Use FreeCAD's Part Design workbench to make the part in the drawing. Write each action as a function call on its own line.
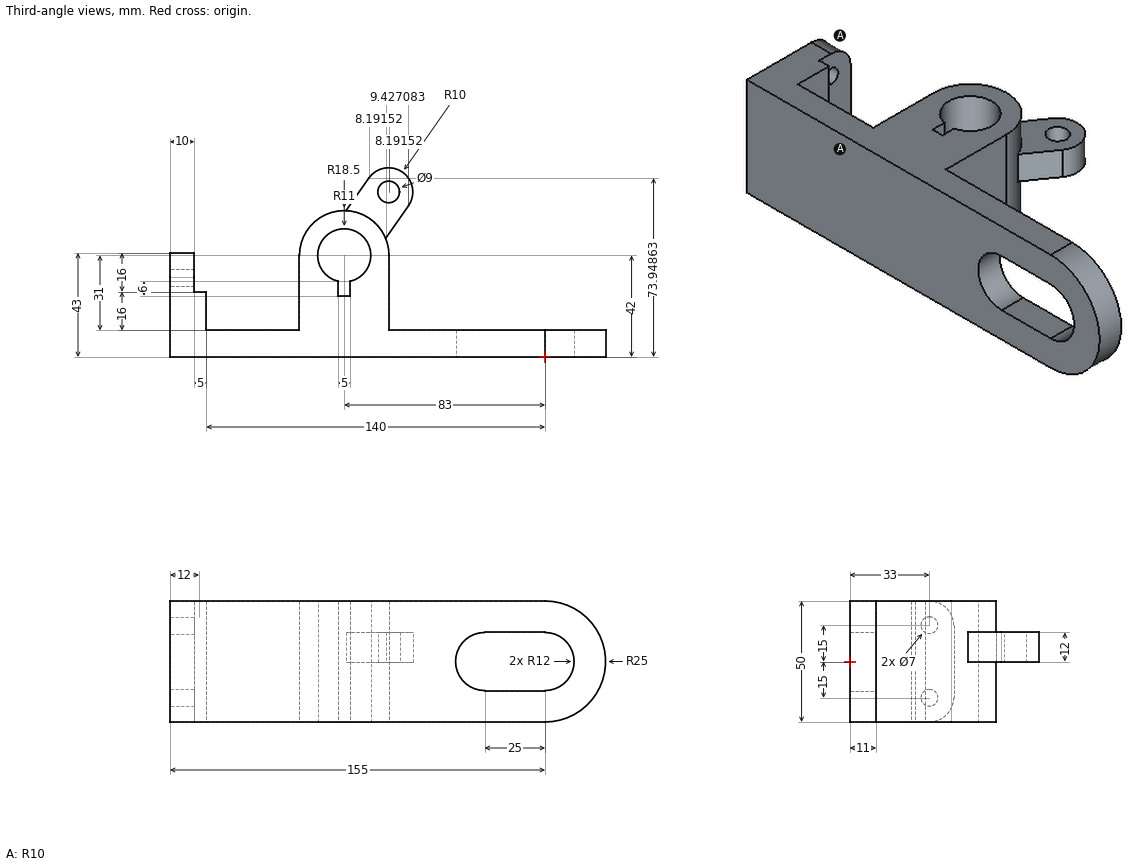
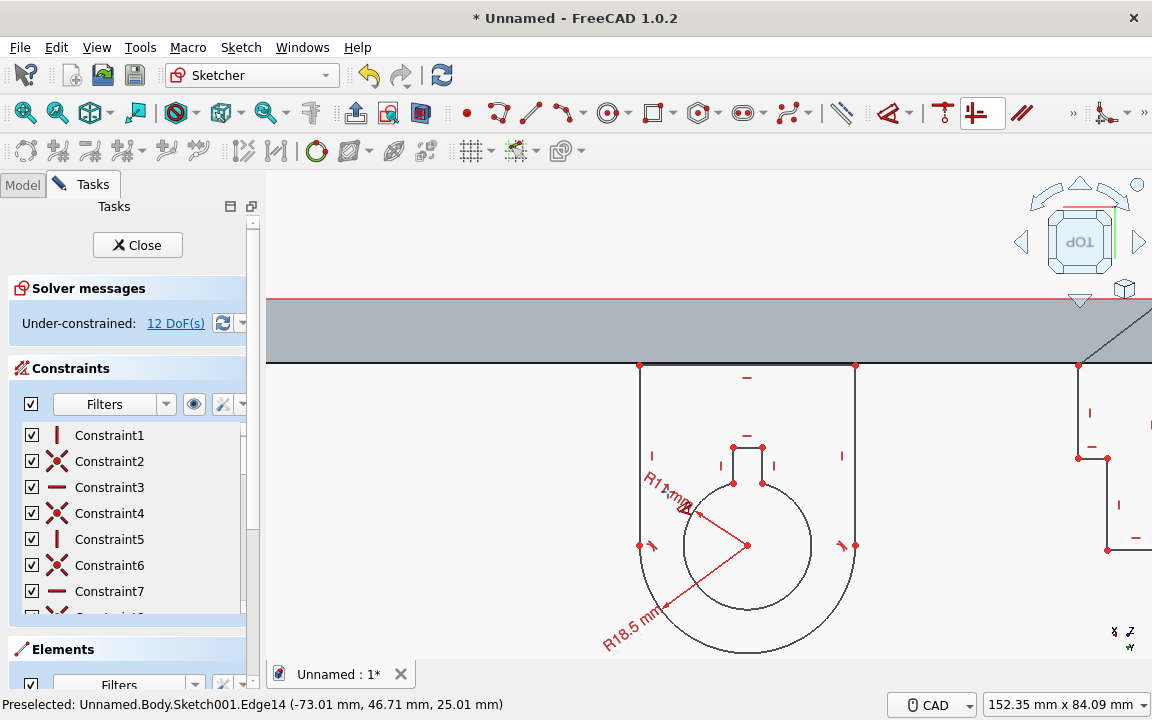
scroll(550, 341, down, 3)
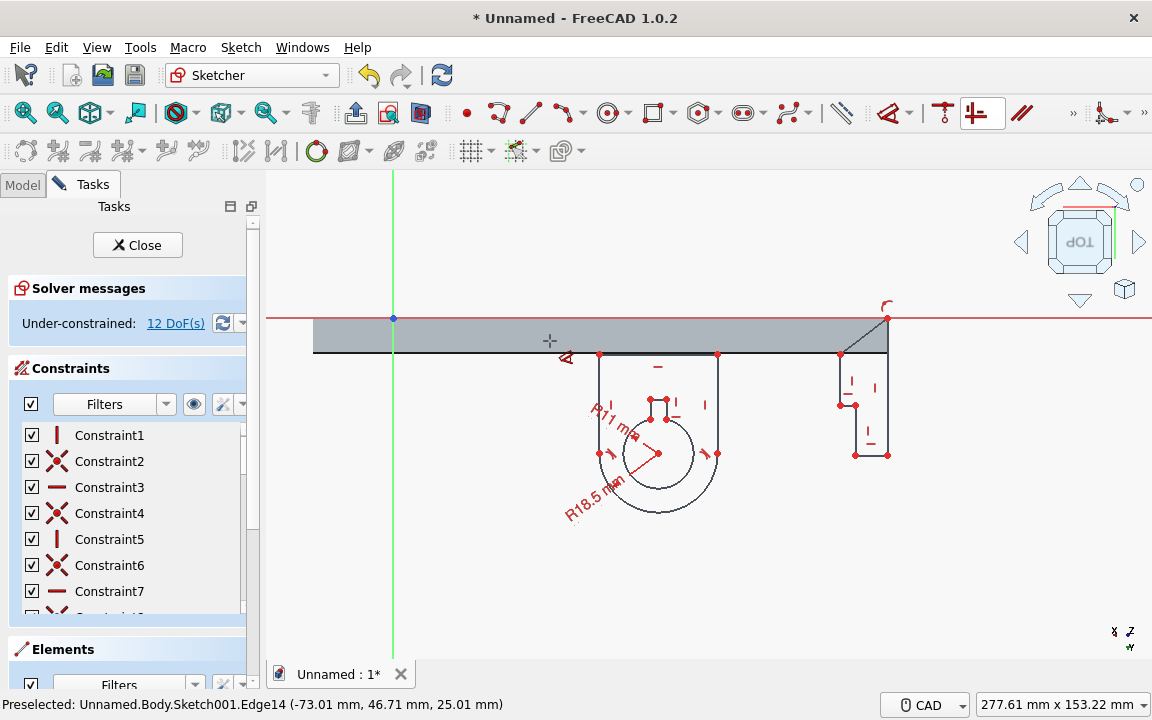
scroll(846, 406, up, 5)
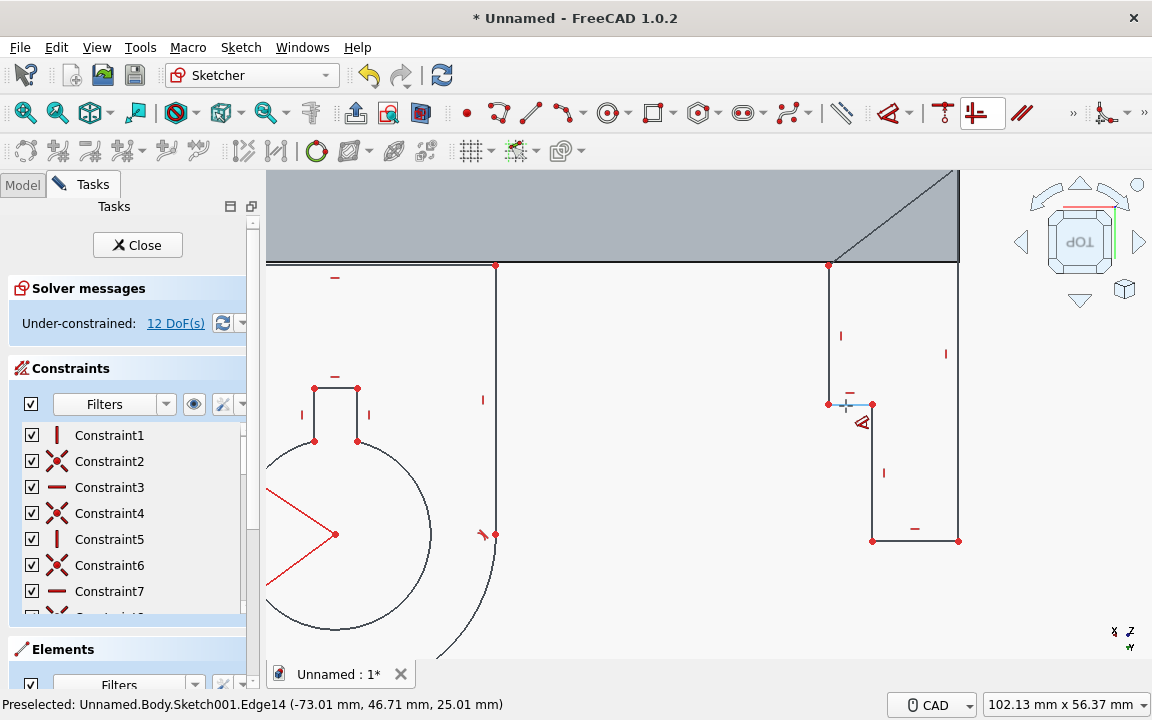
click(846, 405)
click(850, 371)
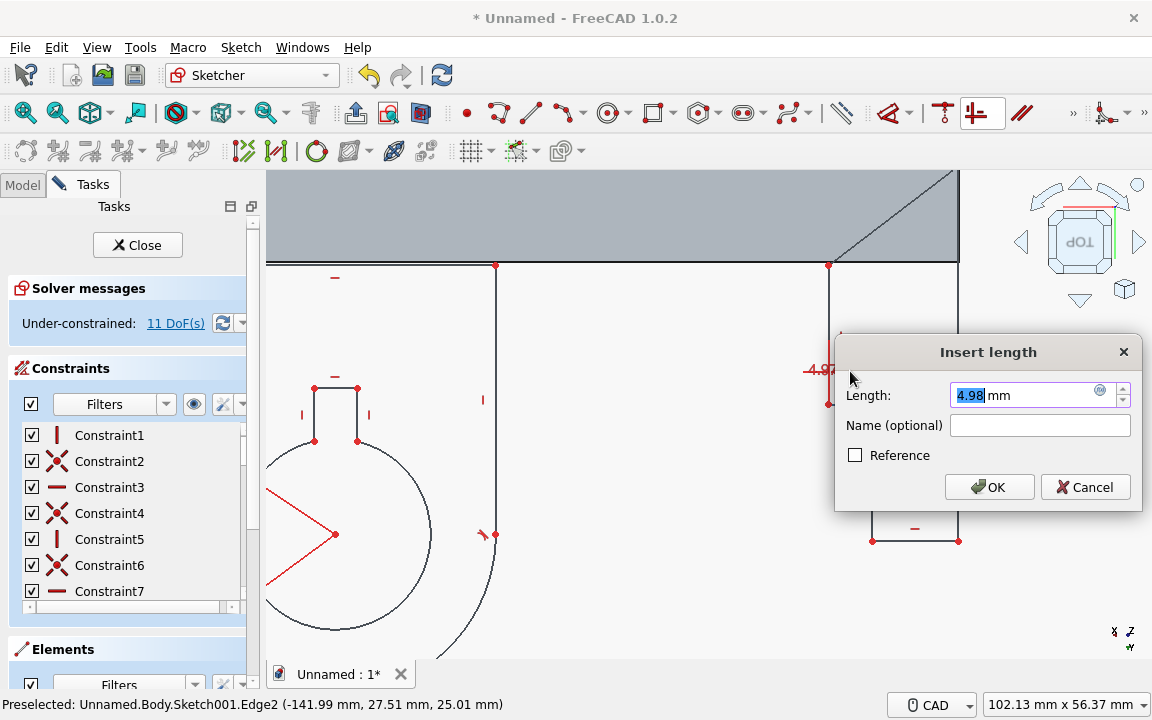
text(5)
key(Return)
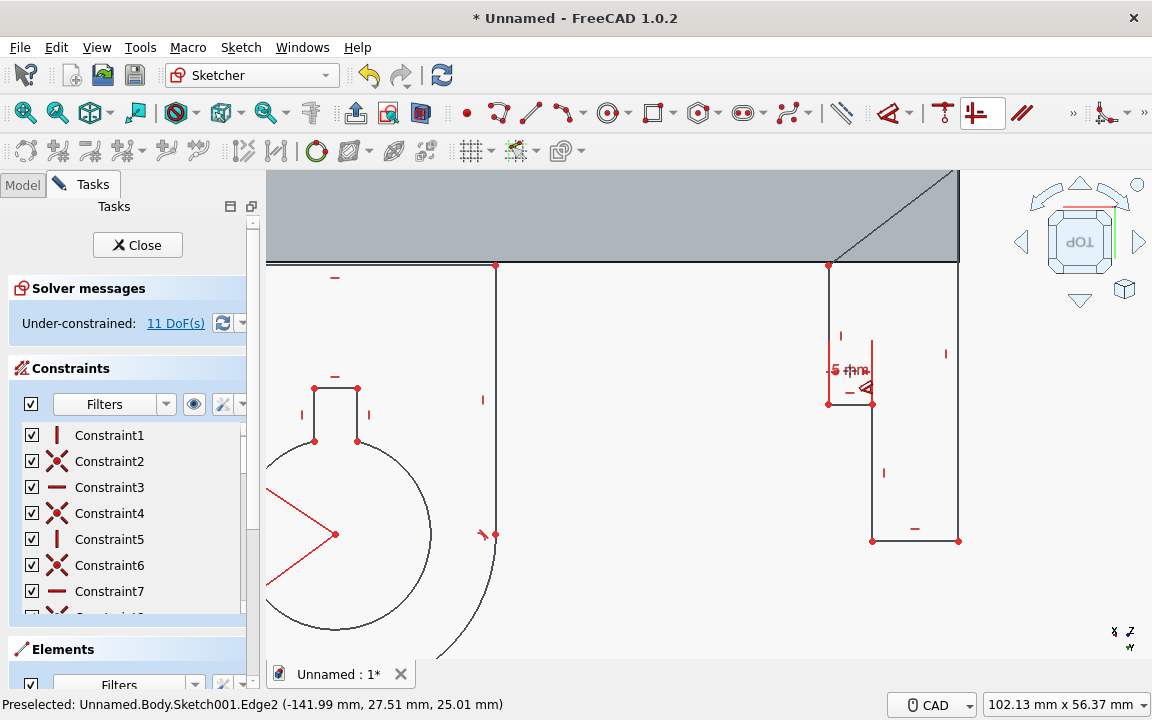
click(314, 425)
click(372, 415)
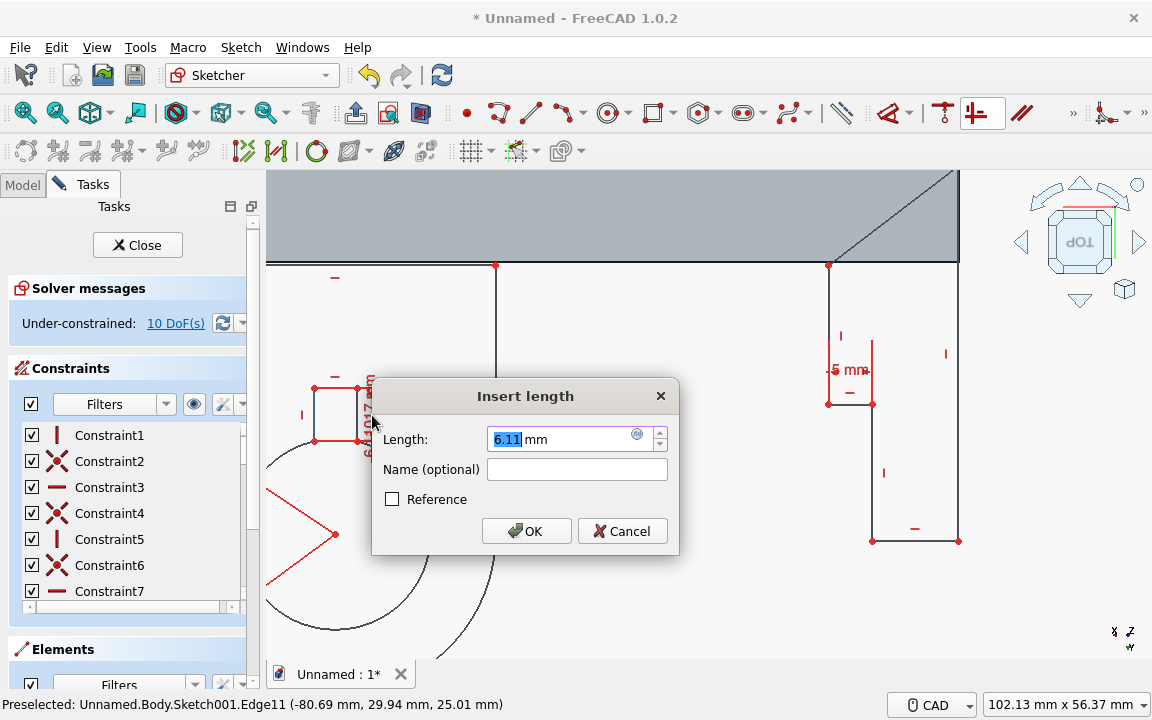
text(6)
key(Return)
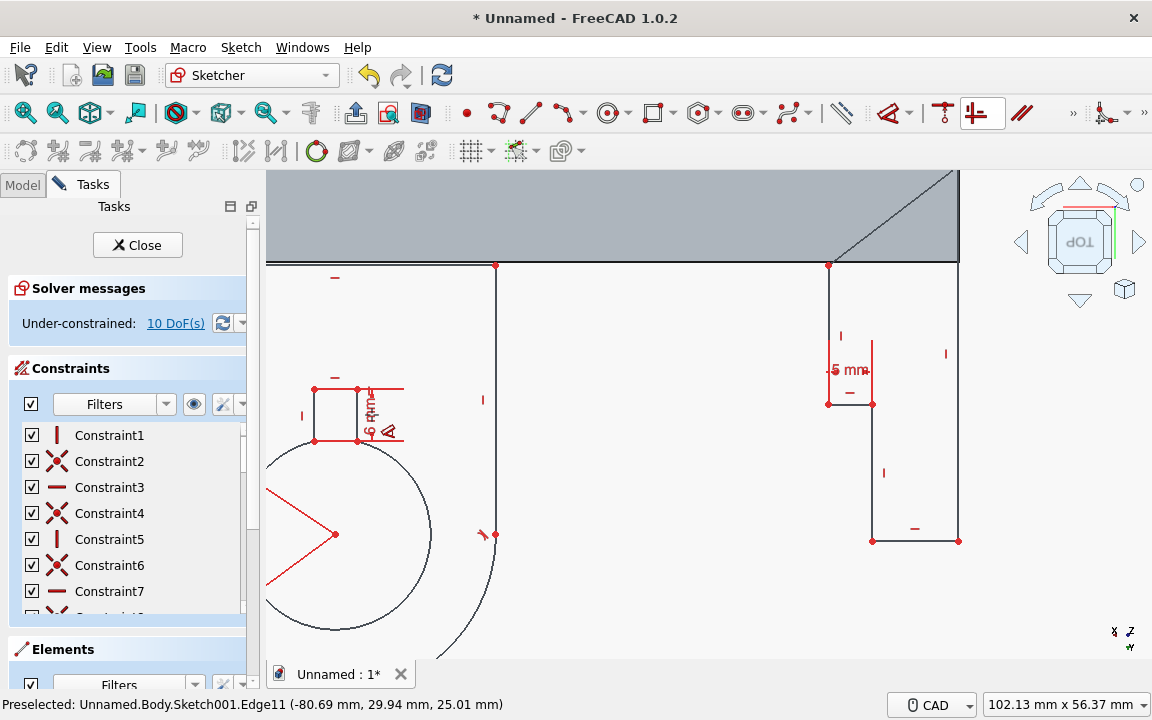
click(327, 389)
click(336, 355)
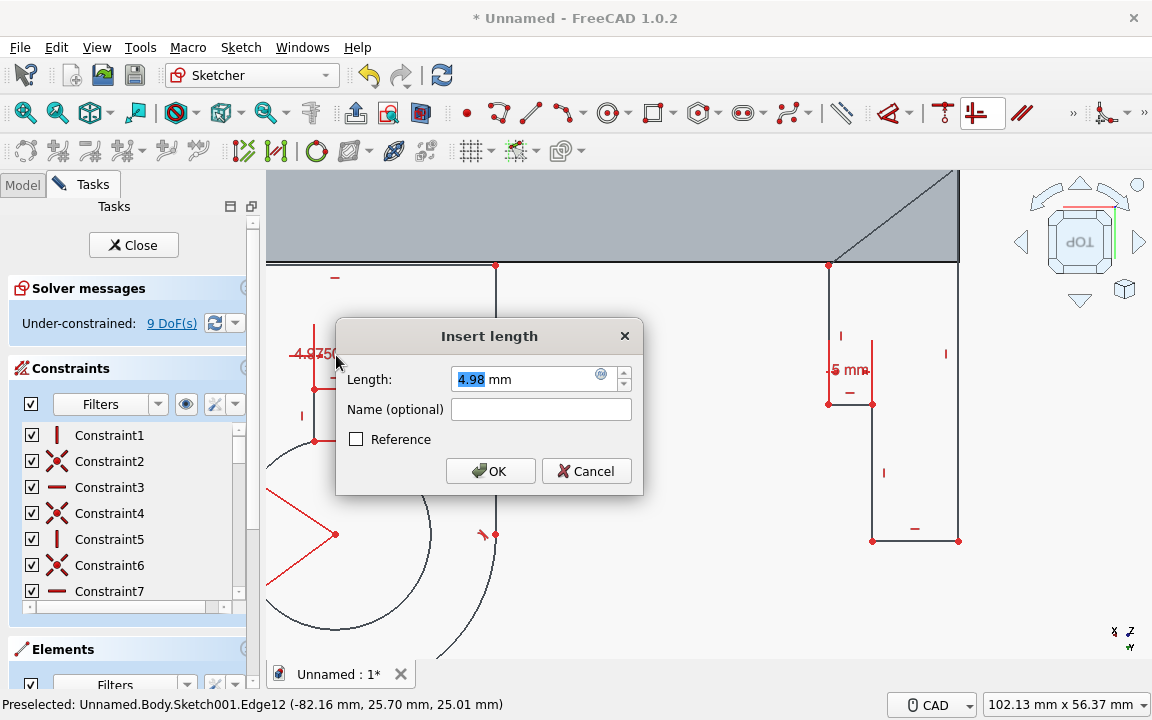
text(5)
key(Return)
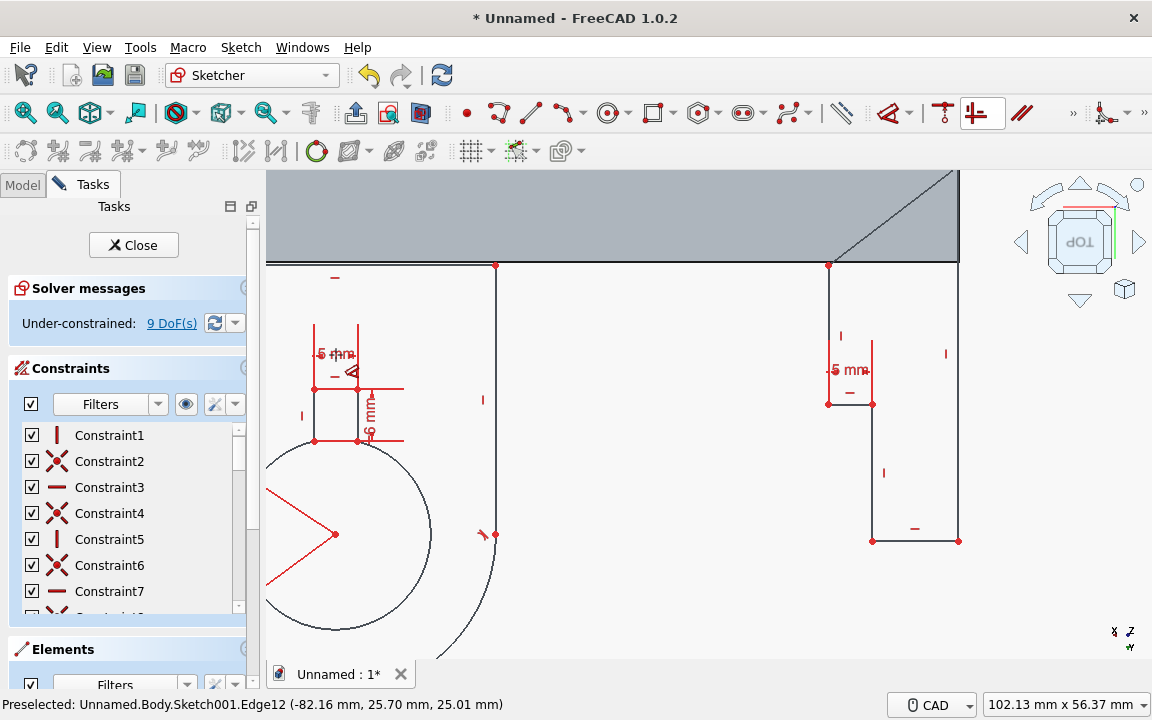
click(358, 405)
click(300, 415)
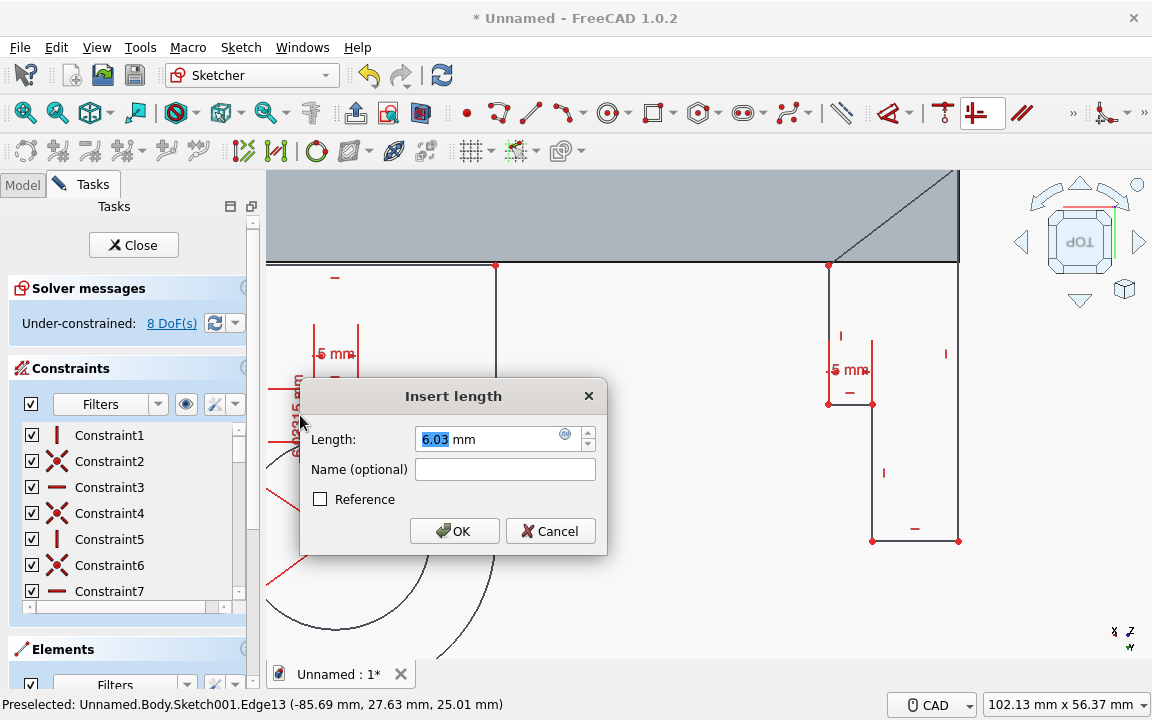
text(6)
key(Return)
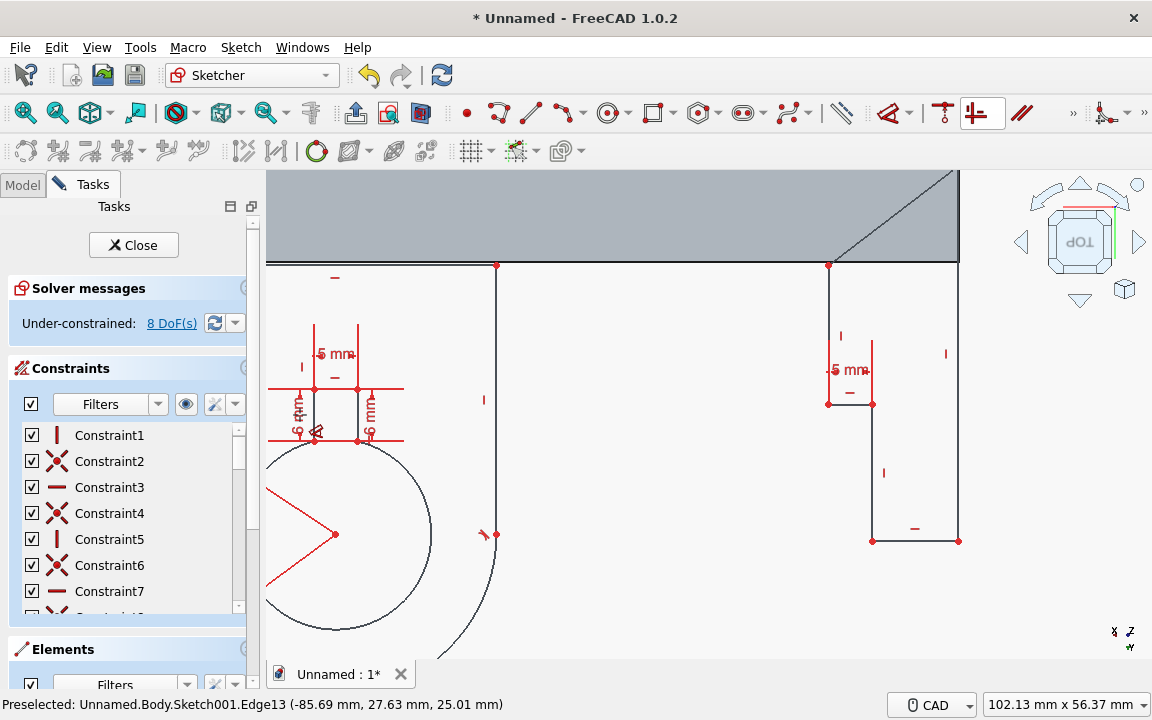
click(829, 307)
click(863, 335)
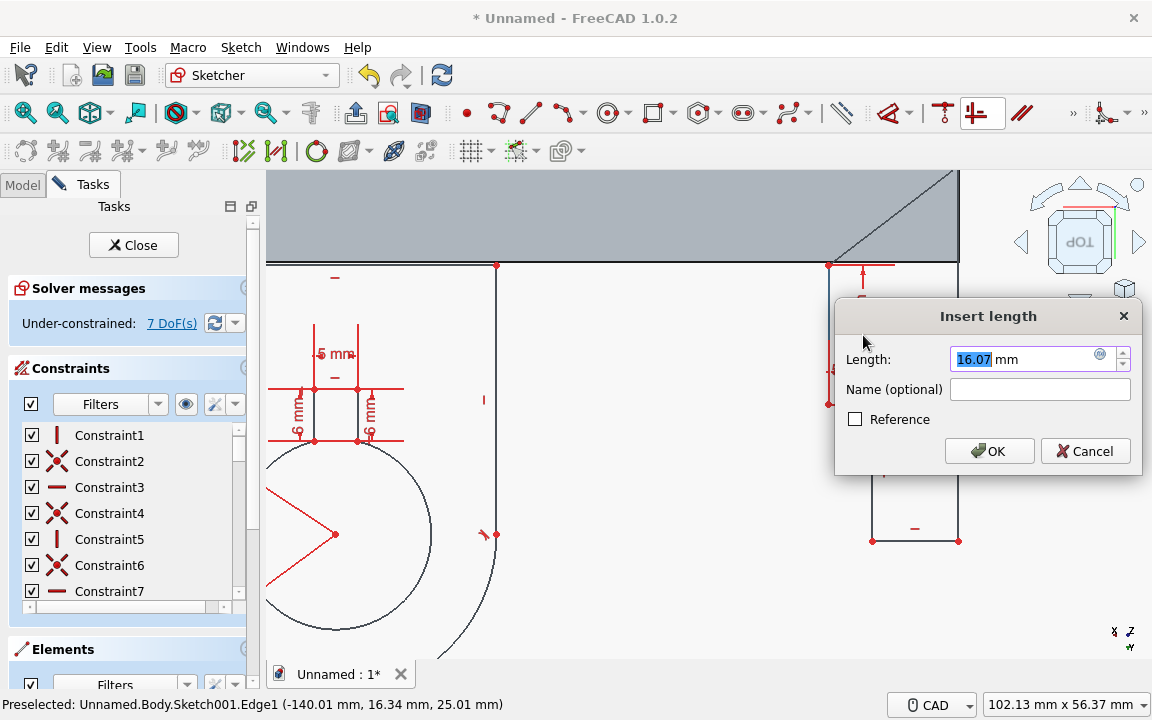
text(16)
key(Return)